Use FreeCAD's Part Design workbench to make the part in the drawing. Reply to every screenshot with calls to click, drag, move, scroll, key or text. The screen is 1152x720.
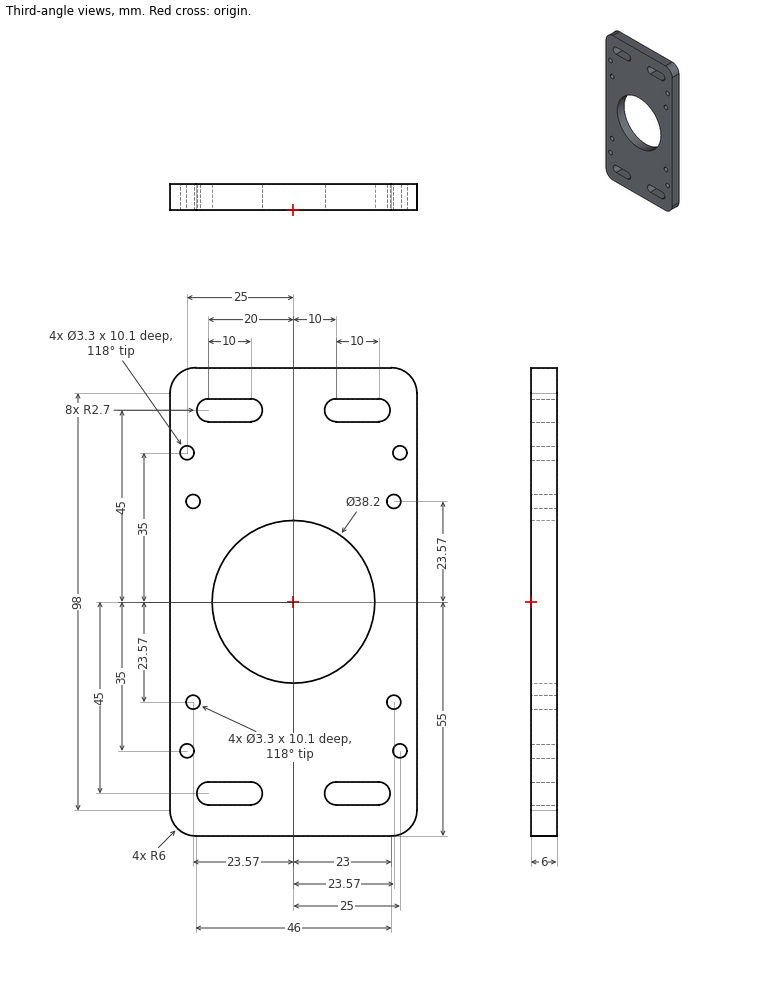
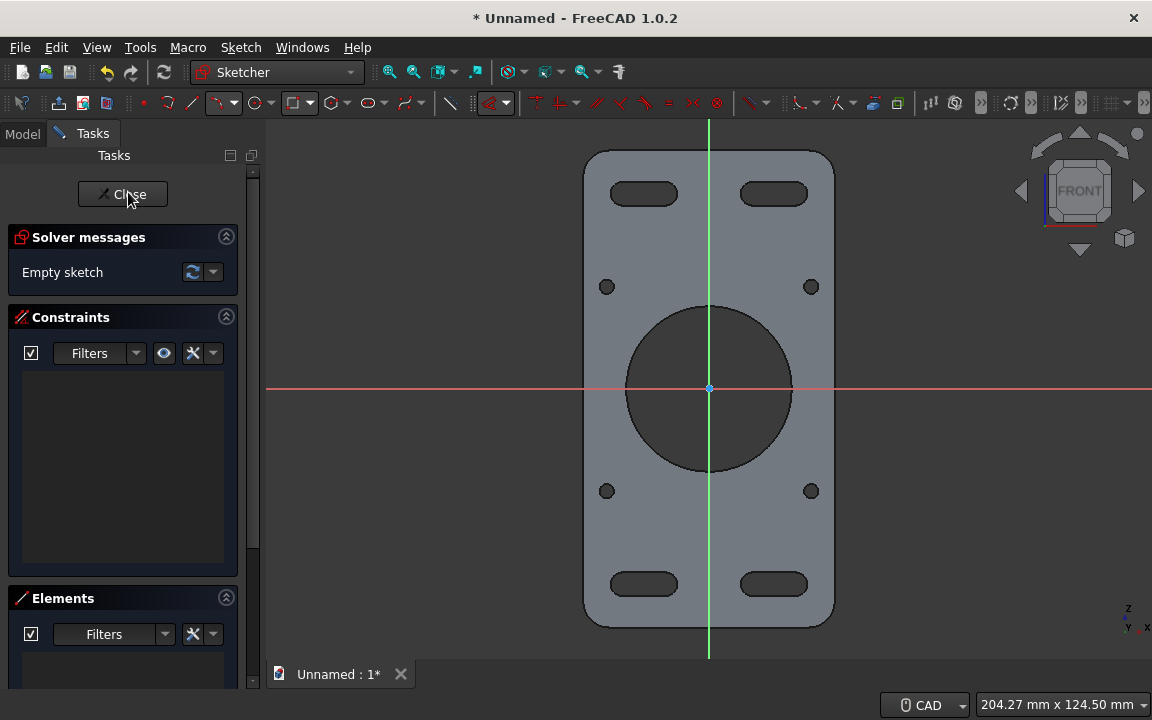
click(256, 104)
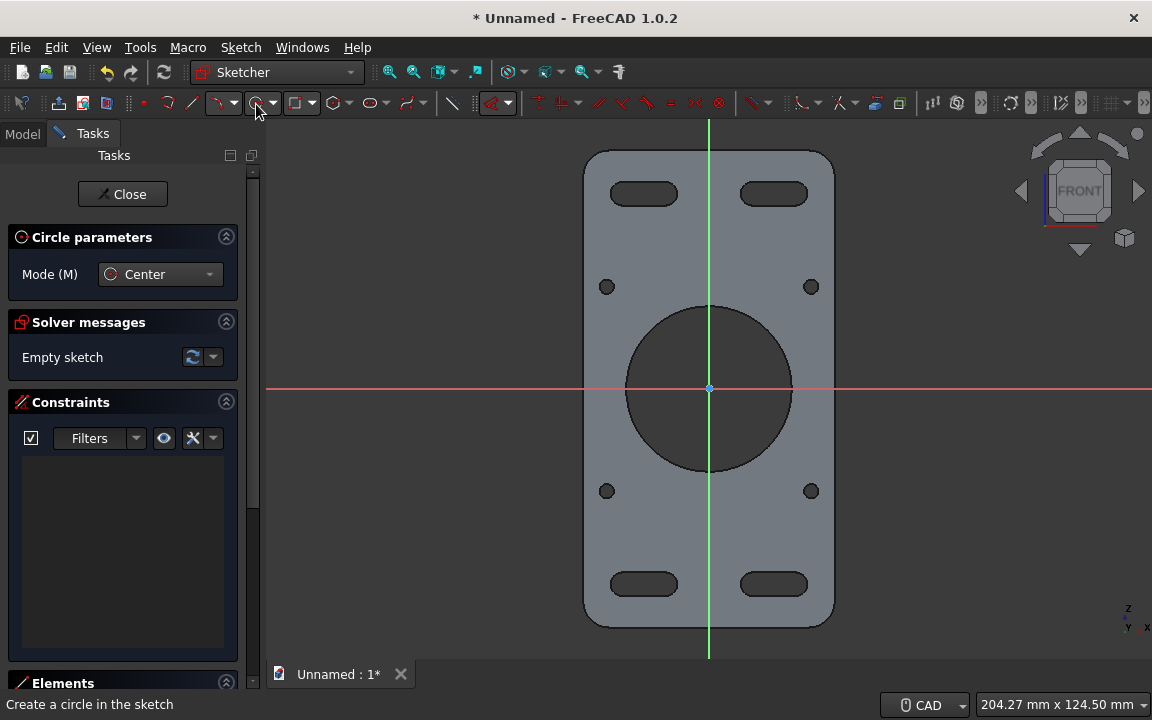
scroll(601, 237, up, 6)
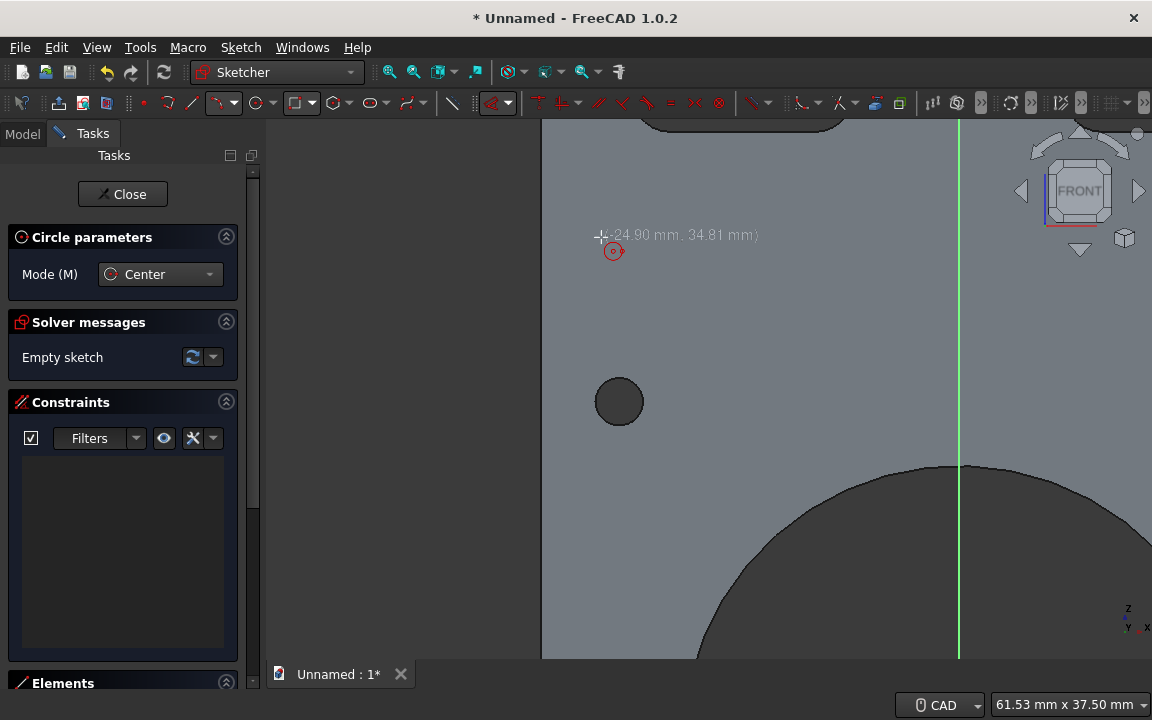
click(599, 237)
move(615, 220)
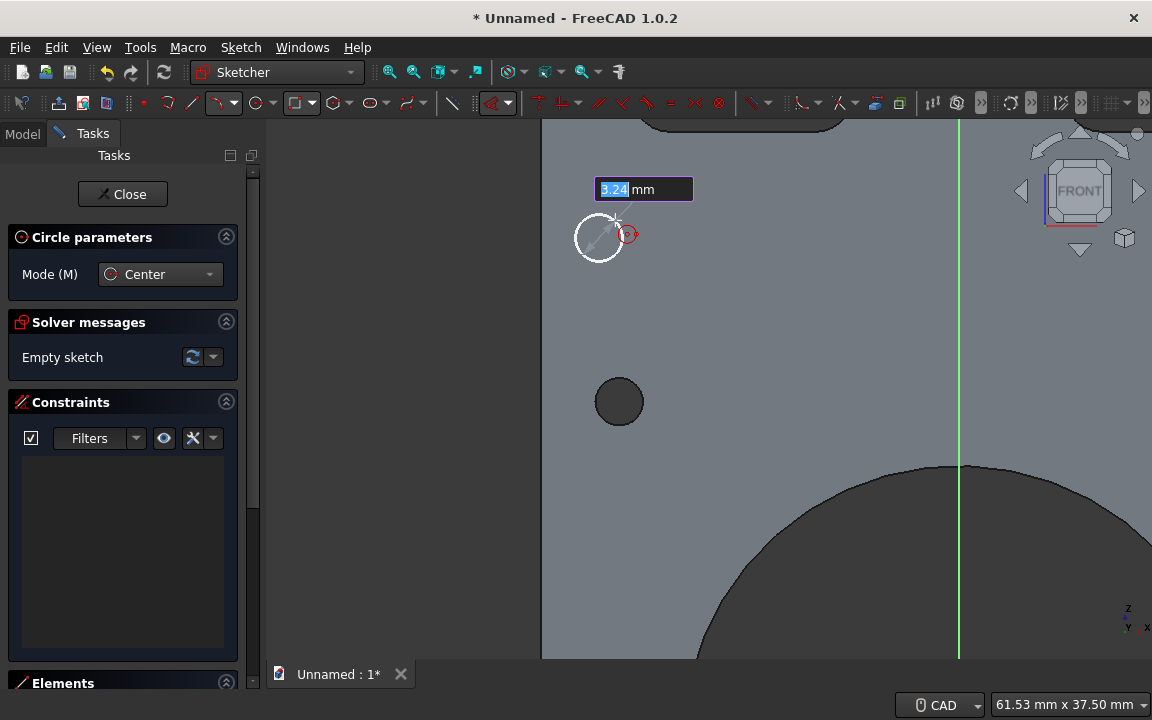
text(3.3)
key(Return)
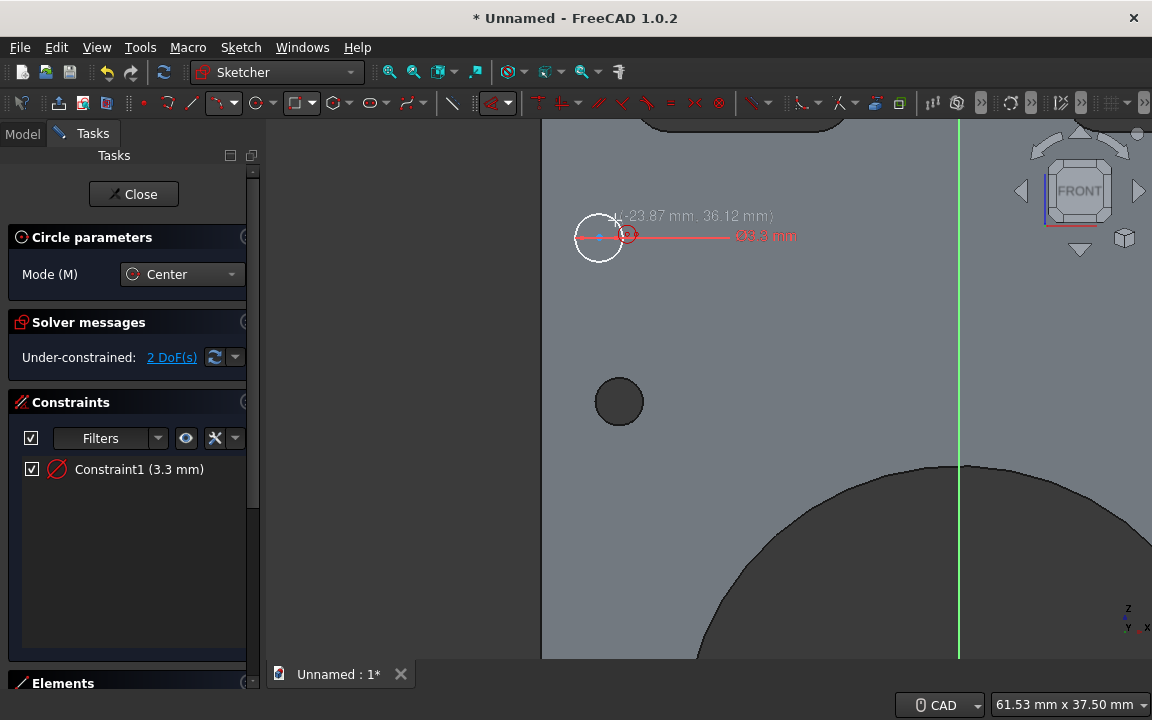
scroll(503, 237, down, 6)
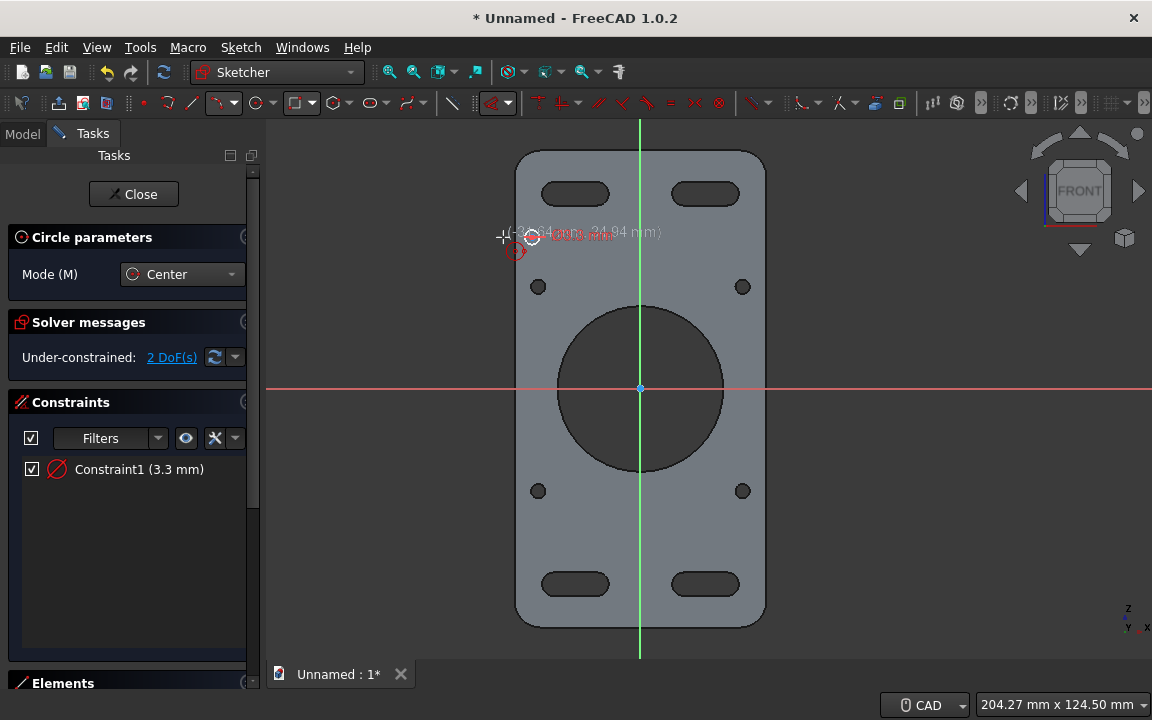
scroll(532, 541, up, 6)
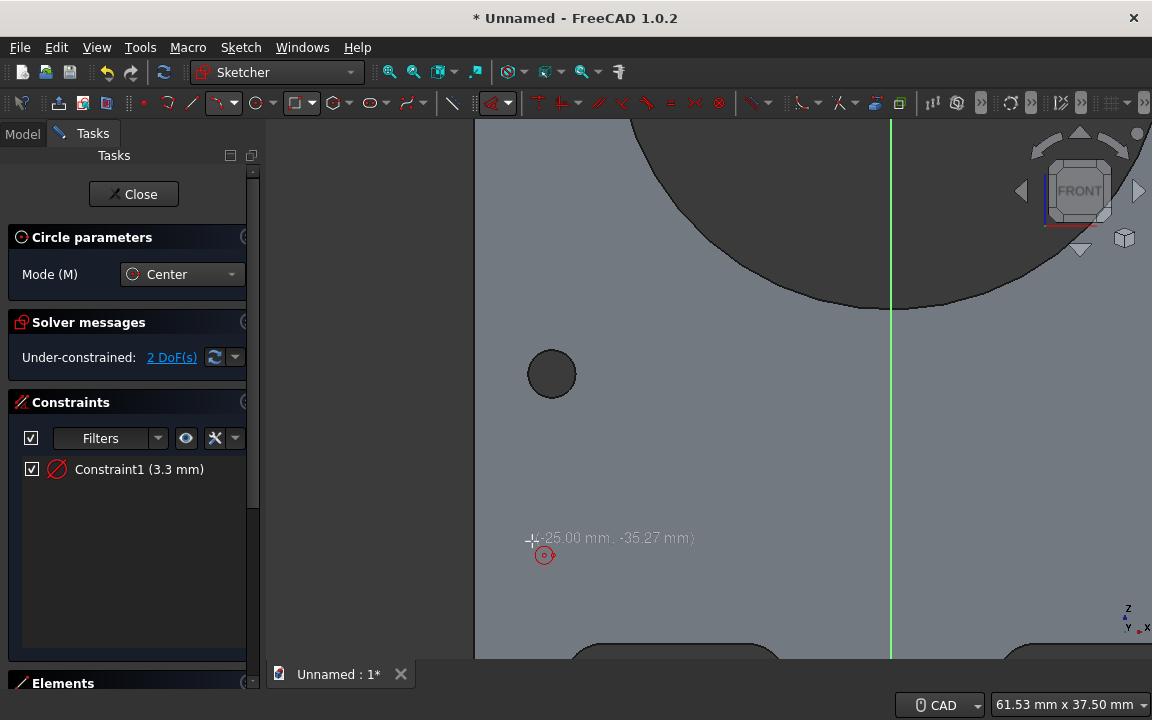
click(531, 539)
move(548, 522)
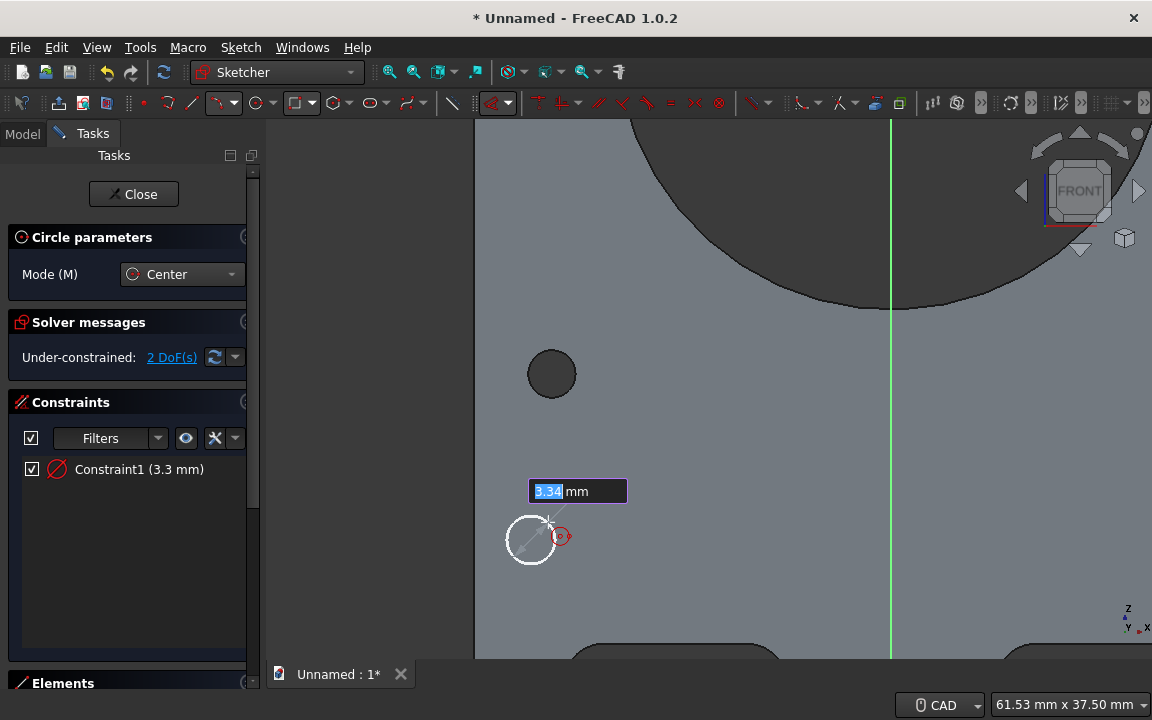
text(3.3)
key(Return)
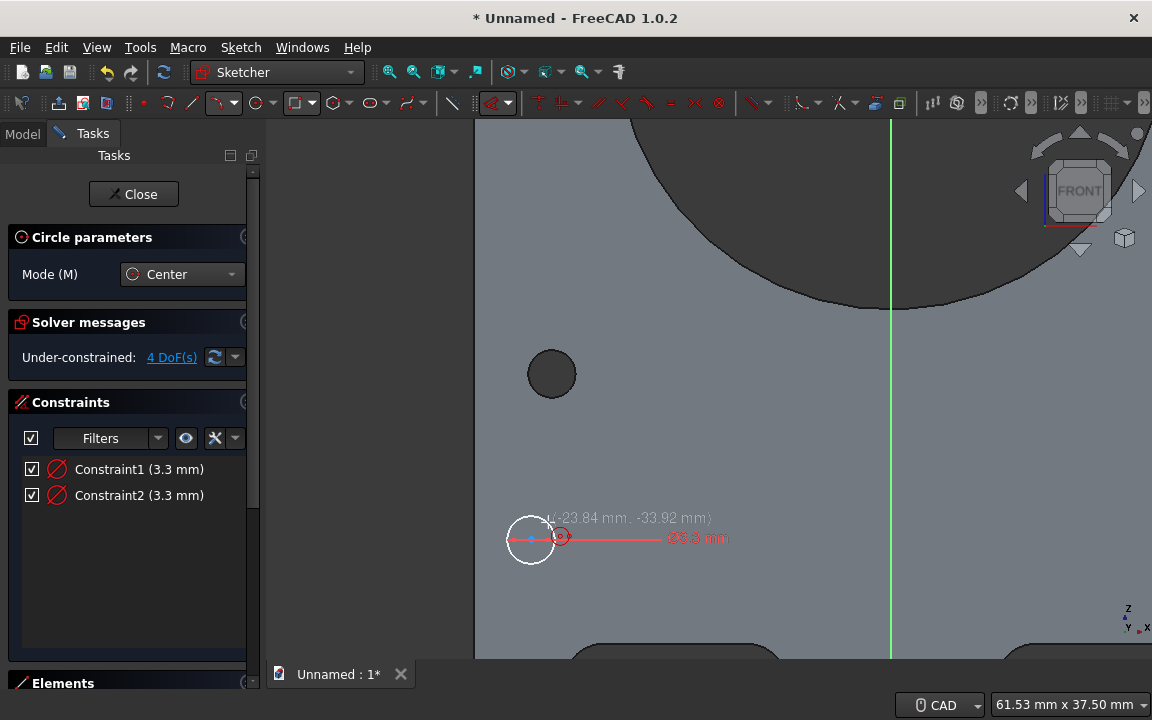
scroll(532, 542, down, 6)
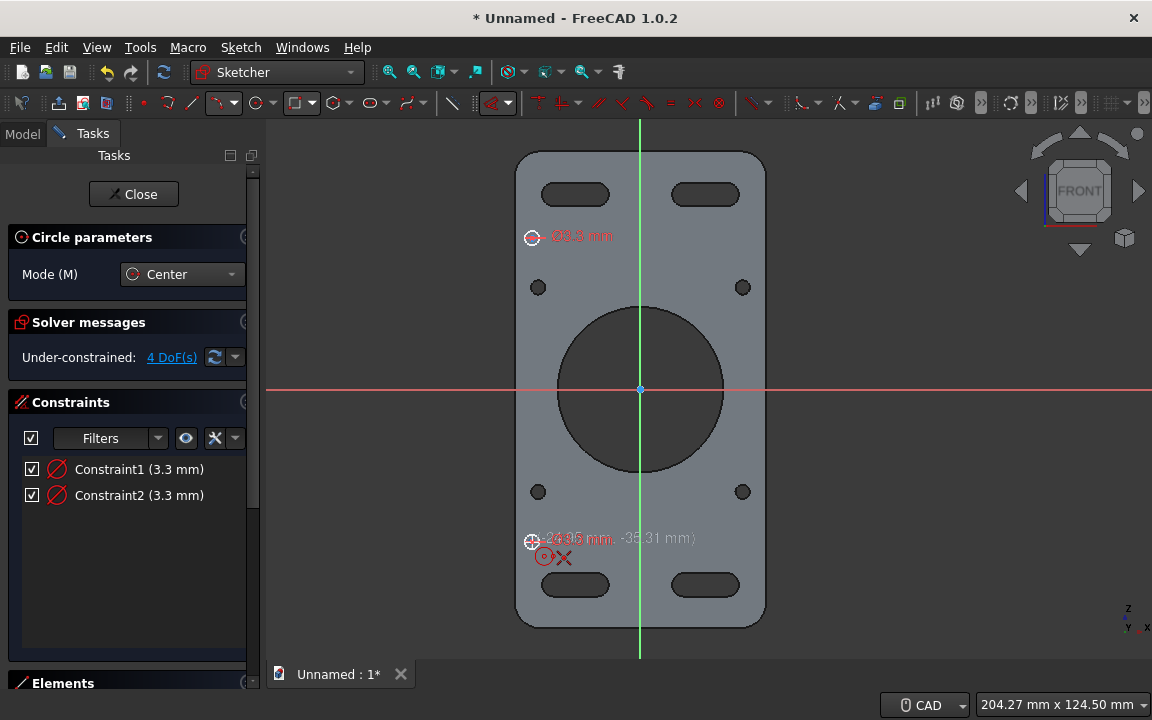
scroll(749, 542, up, 6)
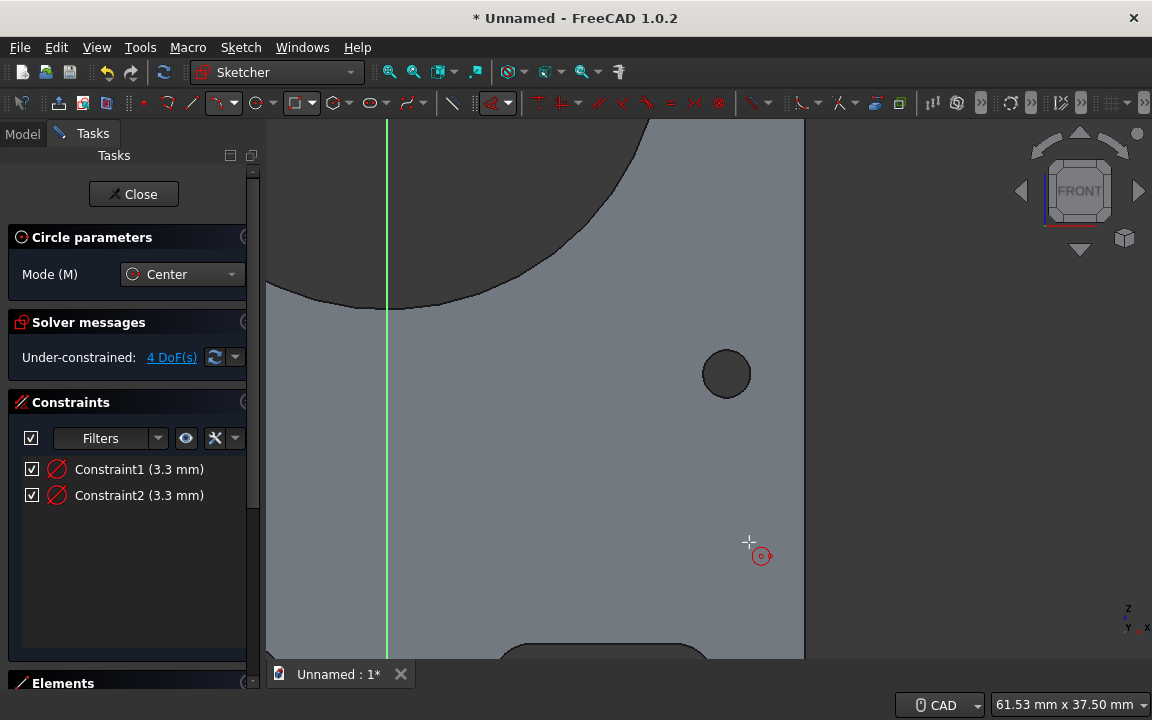
click(747, 539)
move(764, 522)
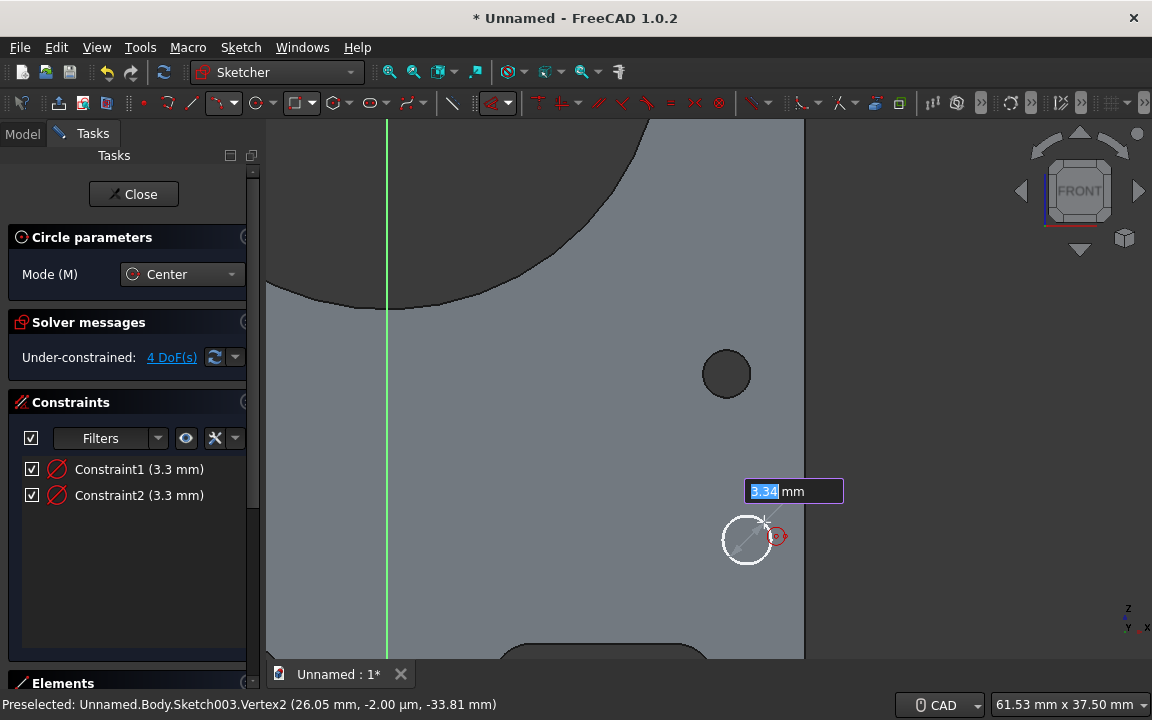
text(3.3)
key(Return)